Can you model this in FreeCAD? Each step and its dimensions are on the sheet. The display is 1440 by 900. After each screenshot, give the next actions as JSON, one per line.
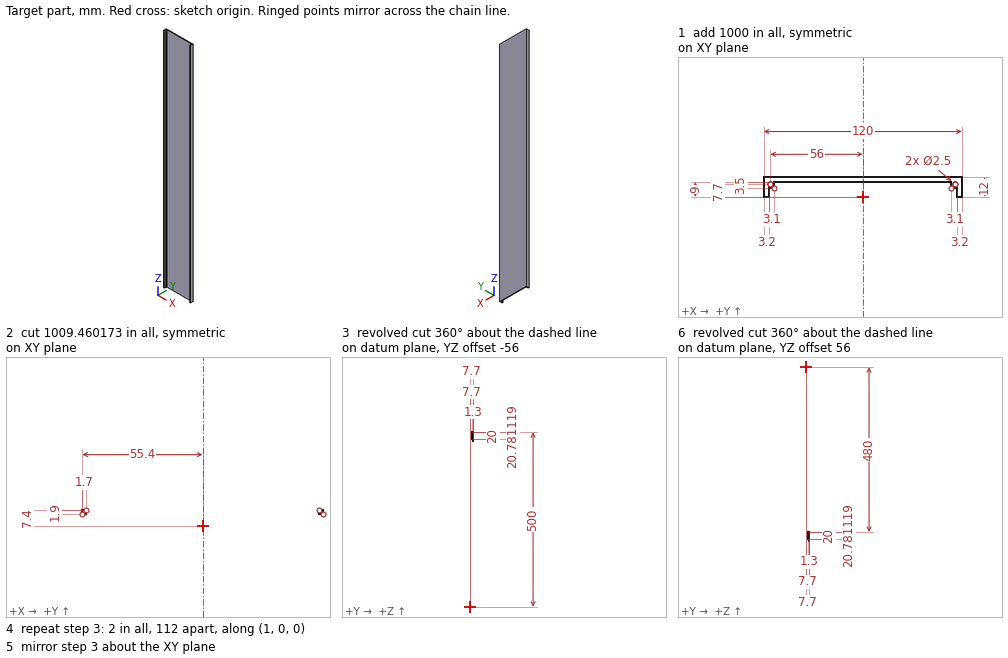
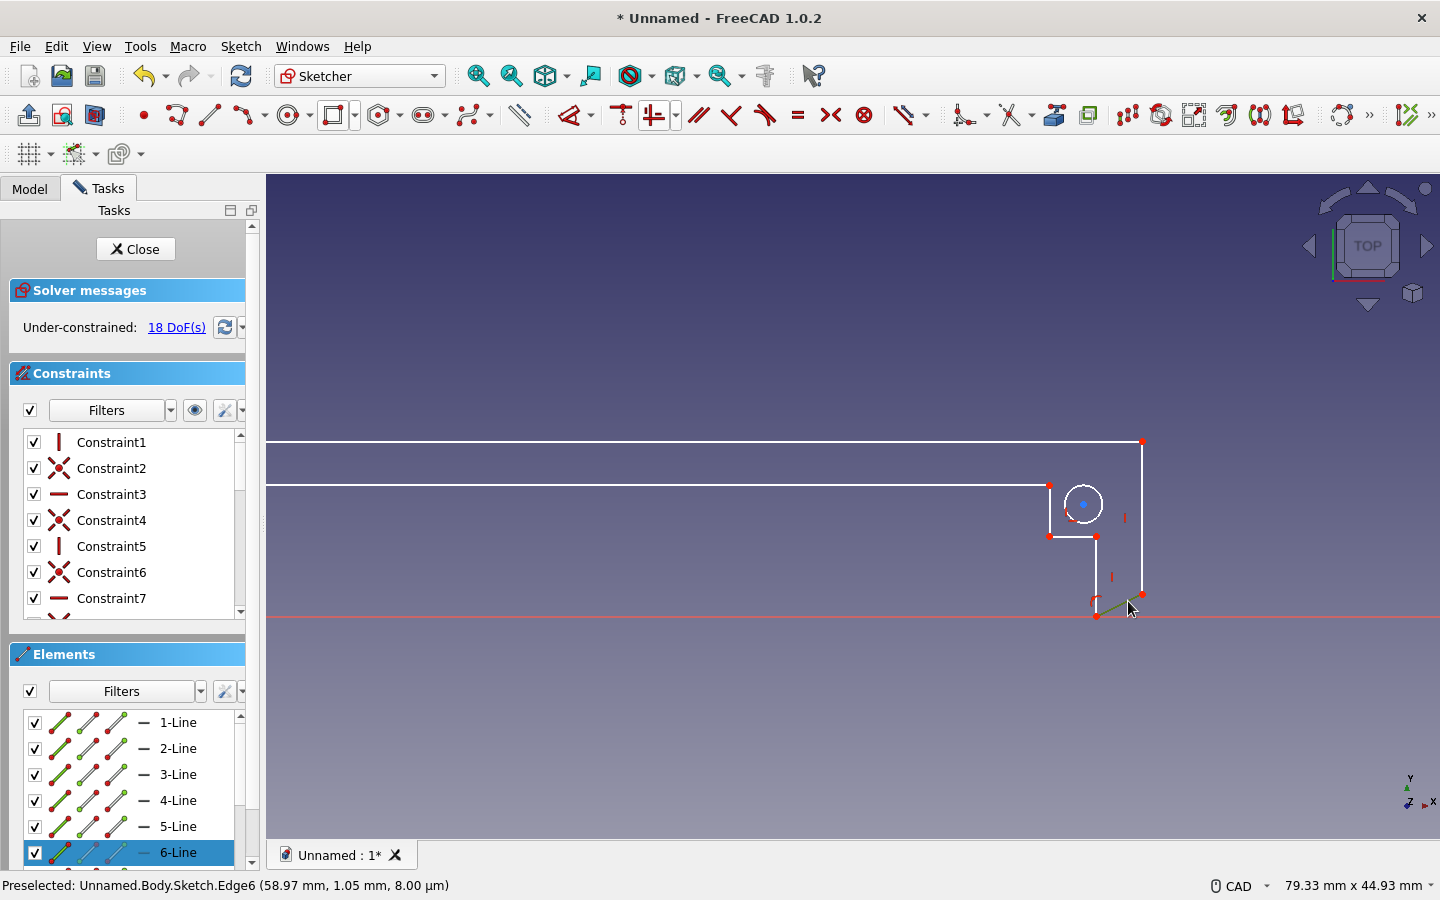
{"action": "key", "text": "h"}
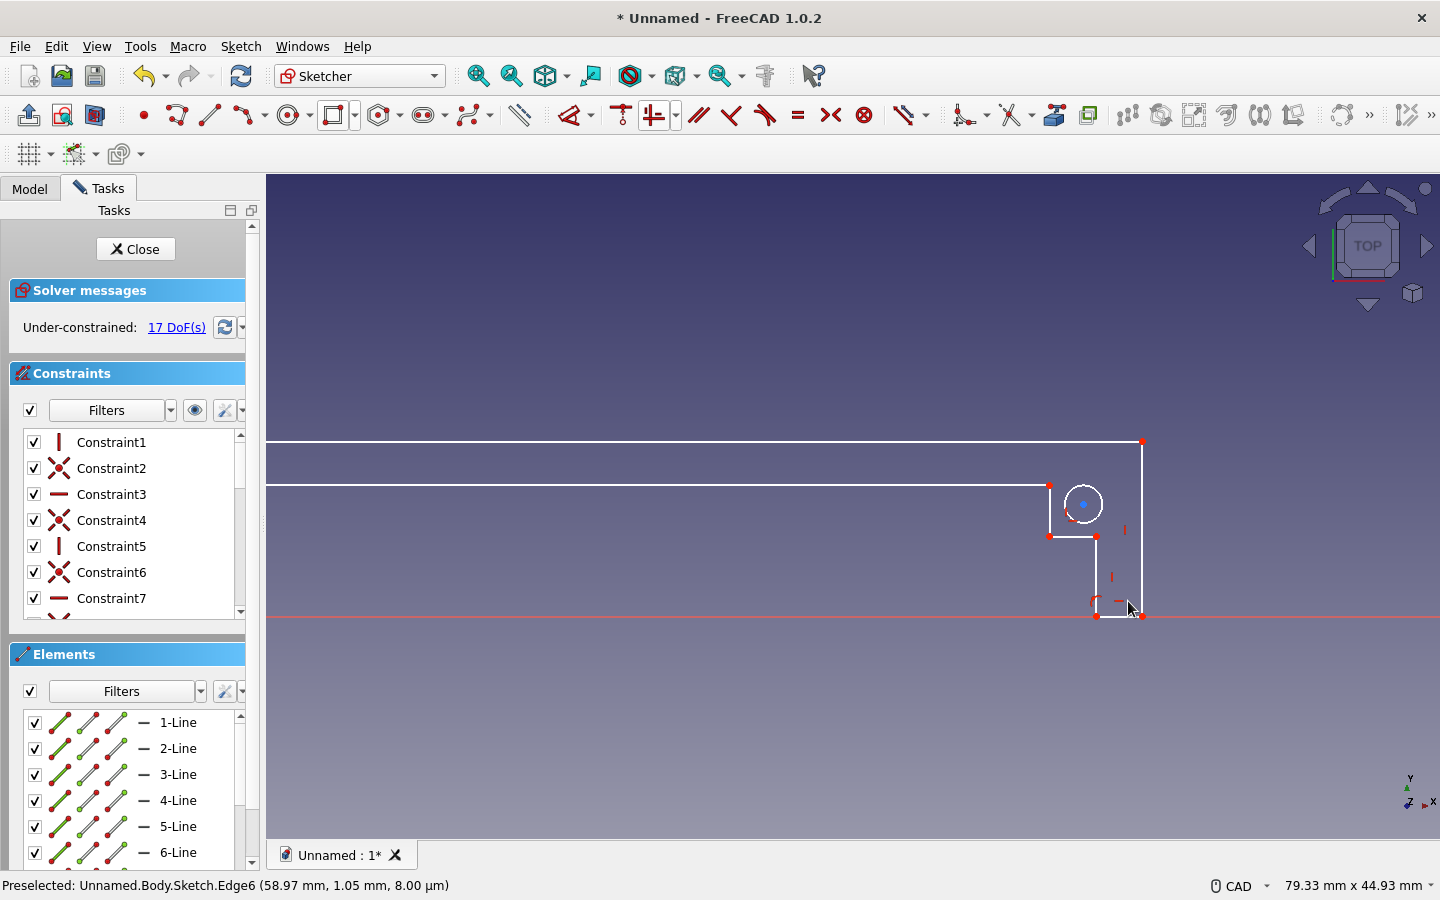
{"action": "scroll", "coordinate": [1093, 494], "scroll_direction": "down", "scroll_amount": 5}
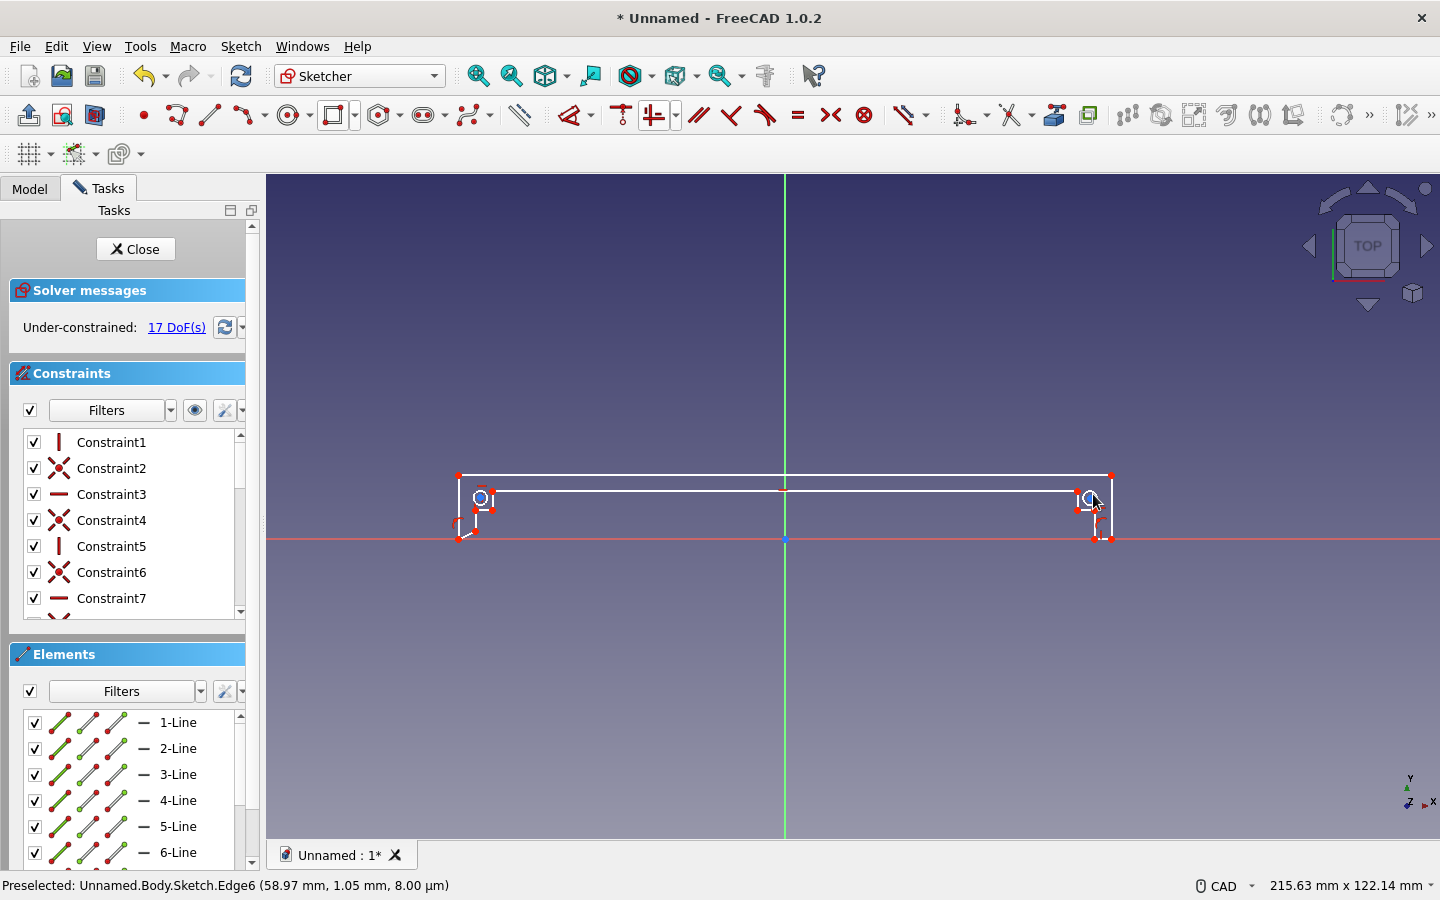
{"action": "scroll", "coordinate": [470, 534], "scroll_direction": "up", "scroll_amount": 5}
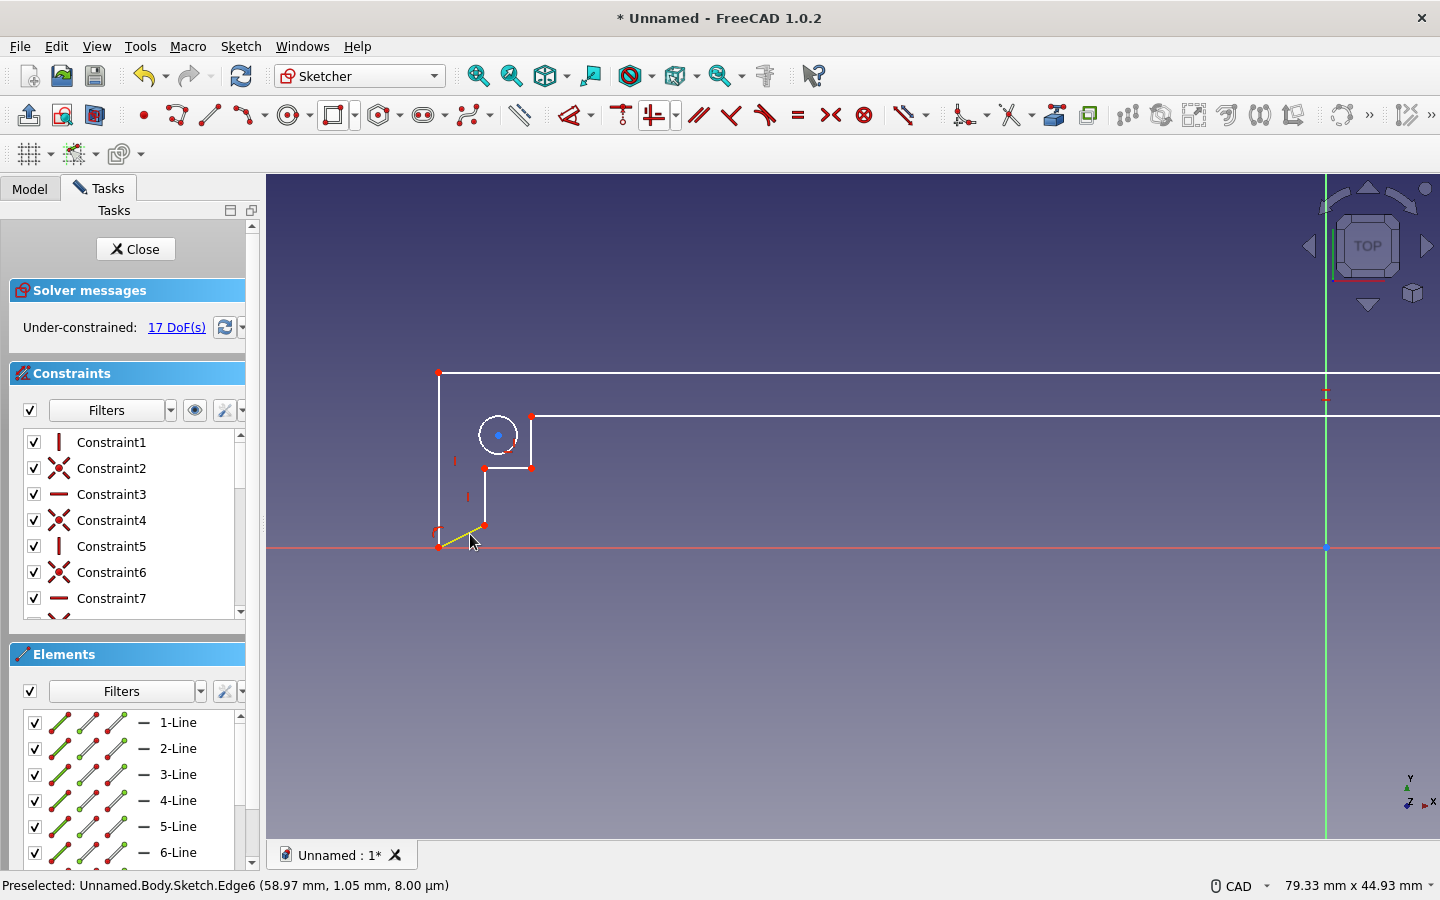
{"action": "left_click", "coordinate": [471, 532]}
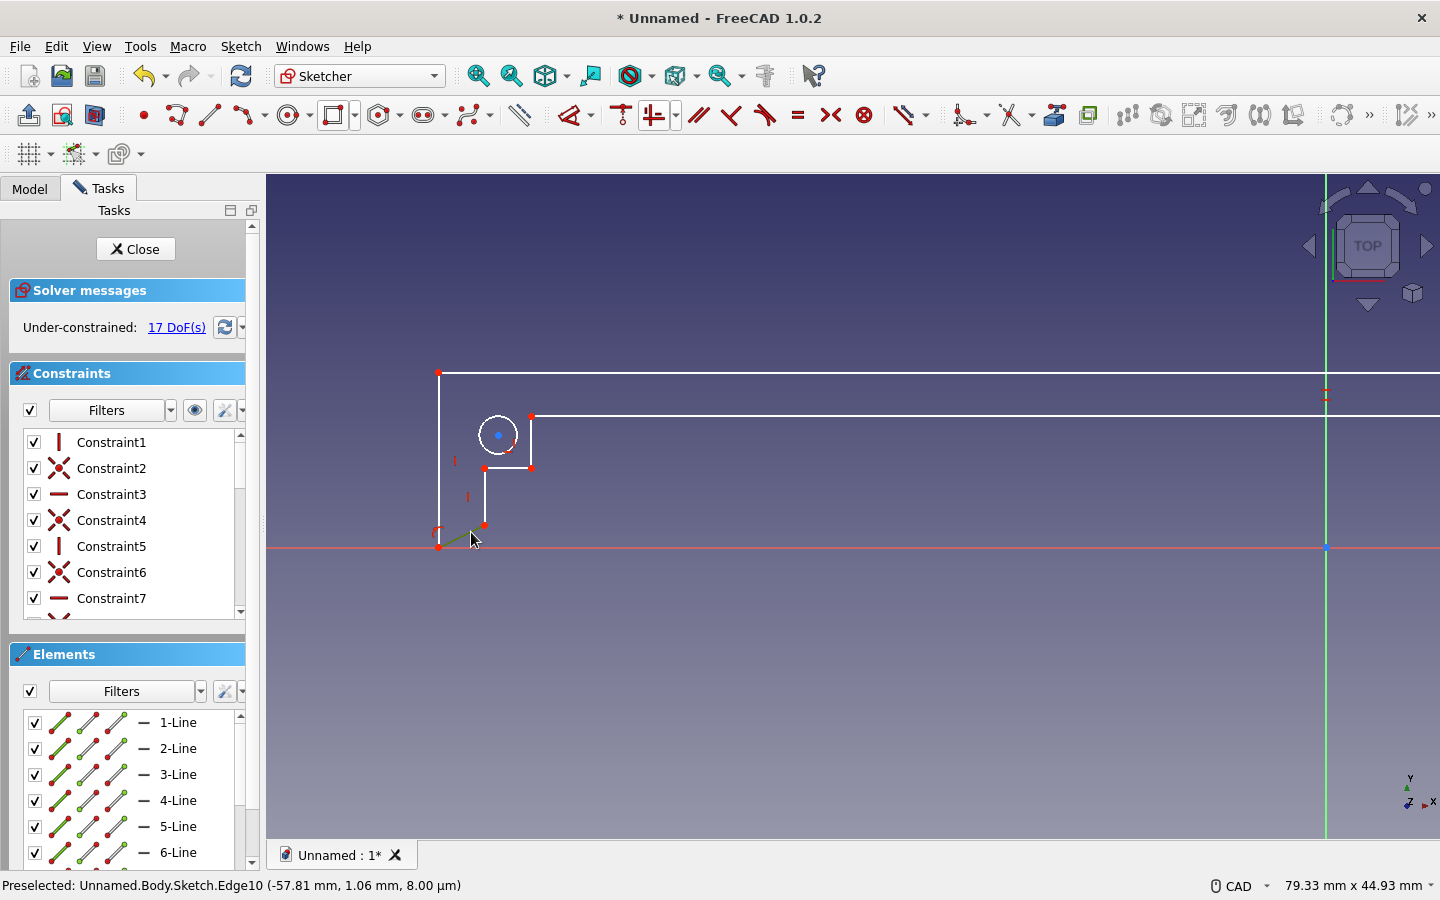
{"action": "key", "text": "h"}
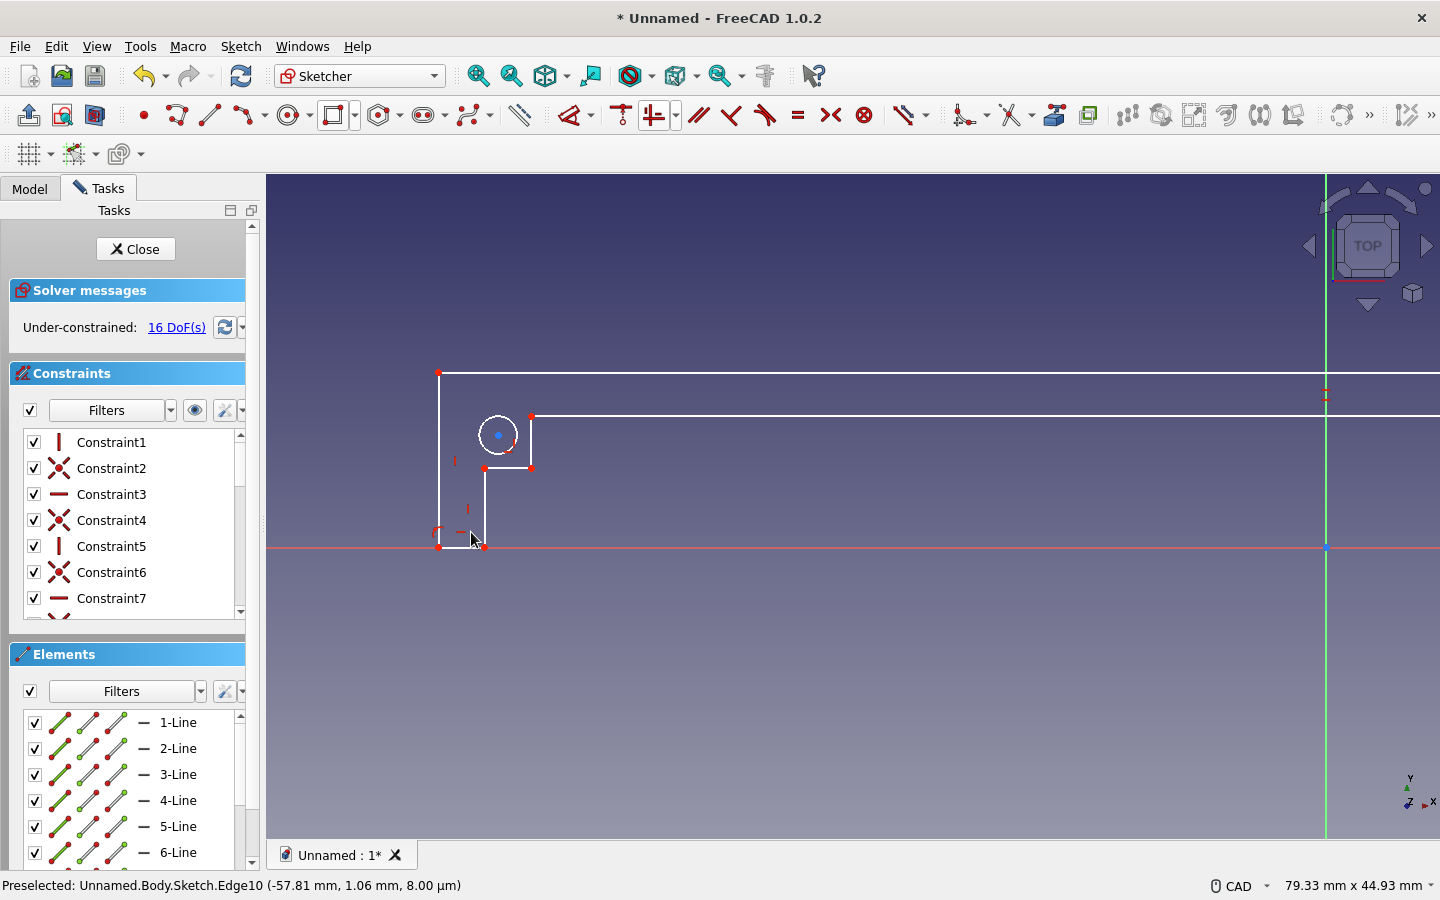
{"action": "left_click", "coordinate": [511, 422]}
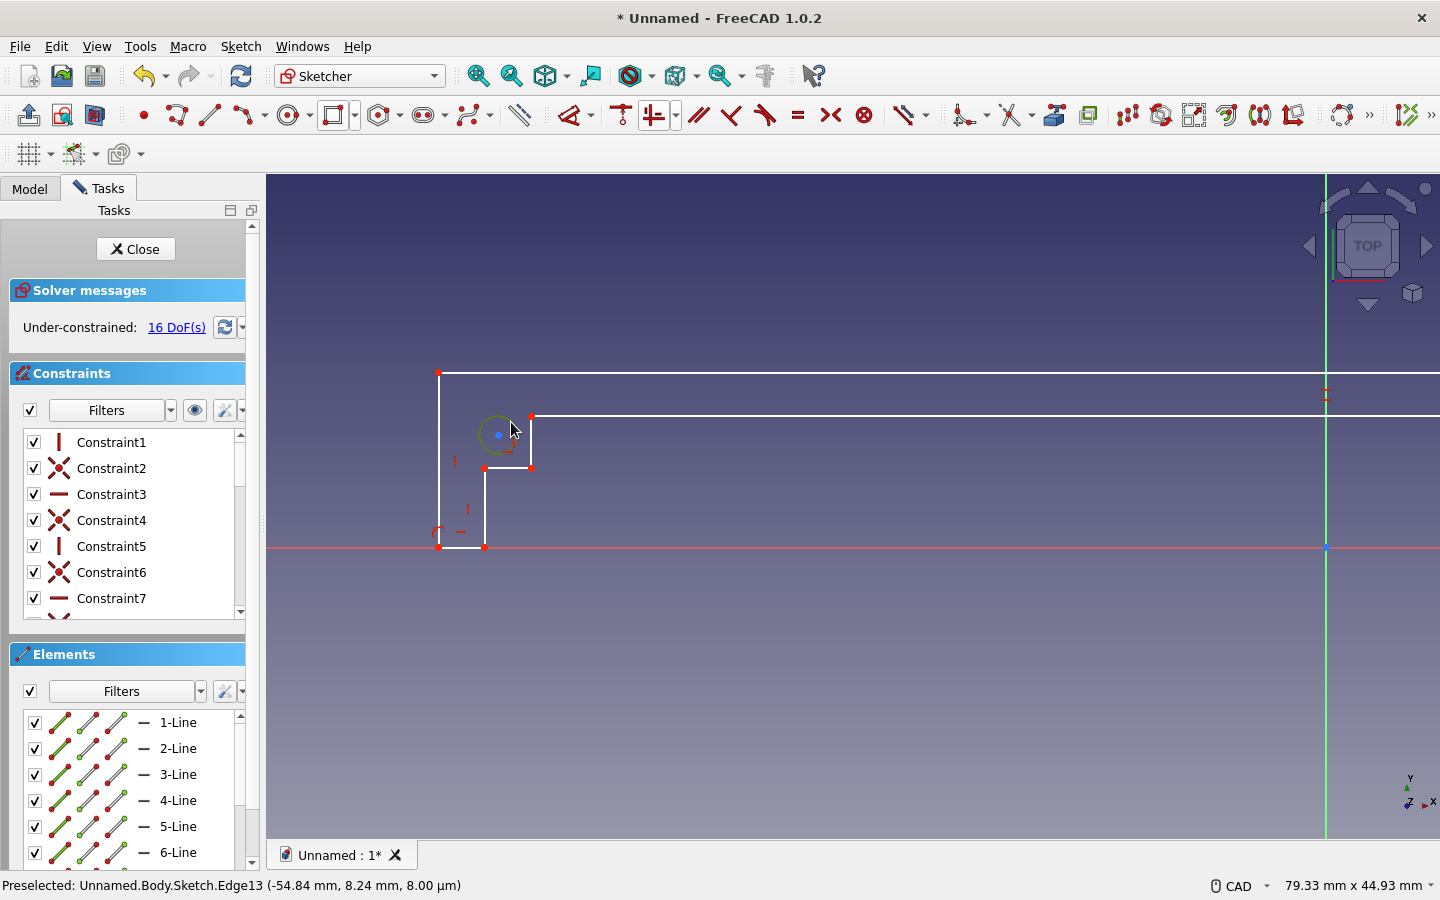
{"action": "scroll", "coordinate": [469, 534], "scroll_direction": "down", "scroll_amount": 5}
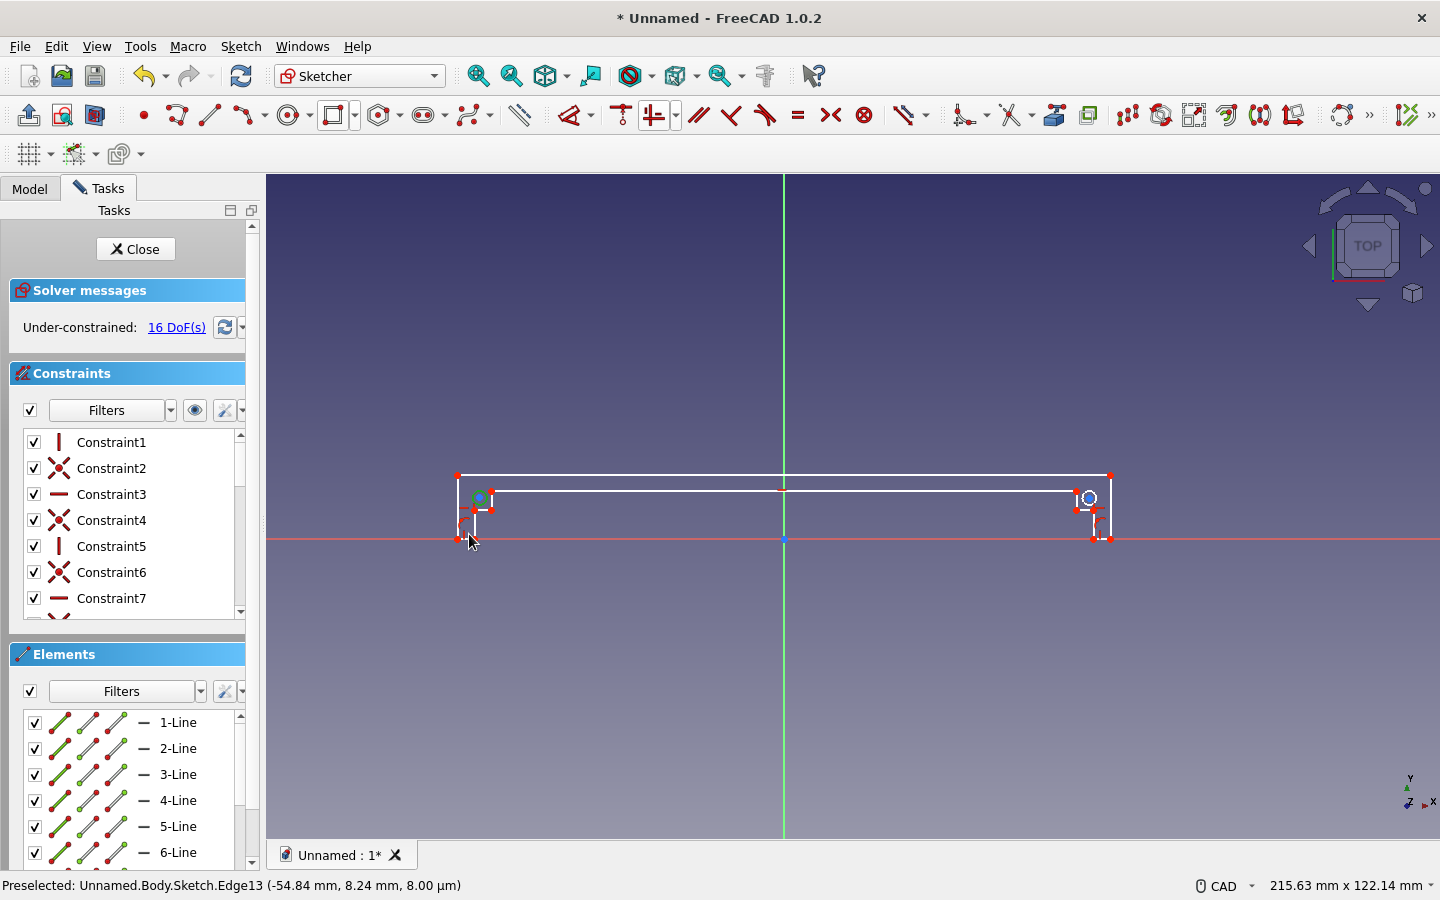
{"action": "scroll", "coordinate": [1094, 493], "scroll_direction": "up", "scroll_amount": 4}